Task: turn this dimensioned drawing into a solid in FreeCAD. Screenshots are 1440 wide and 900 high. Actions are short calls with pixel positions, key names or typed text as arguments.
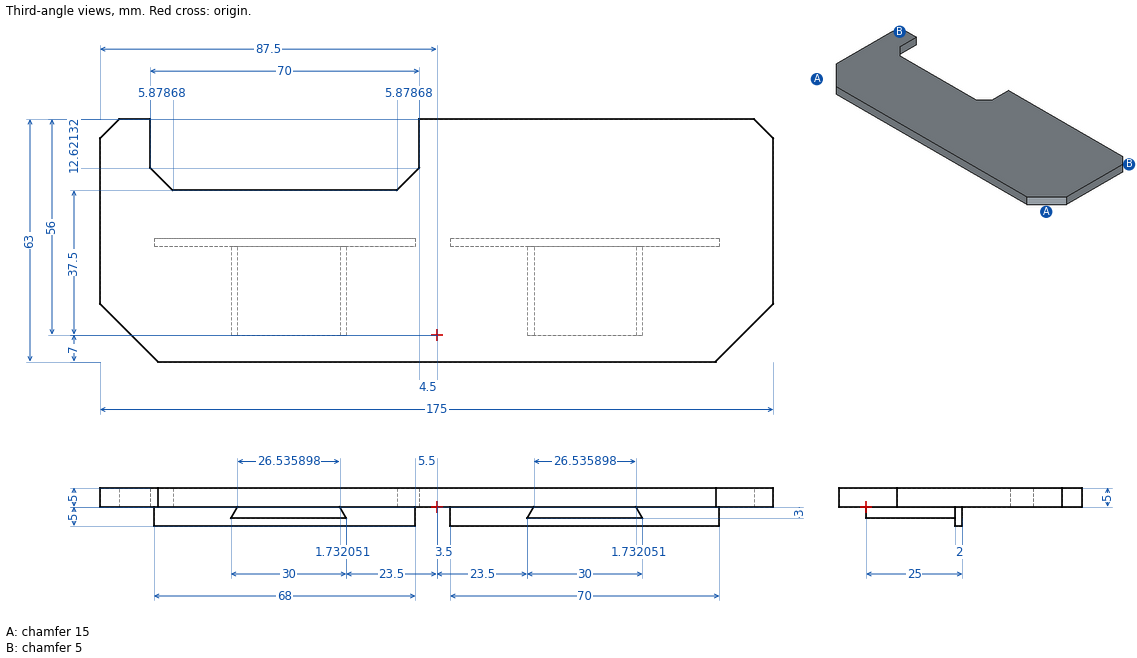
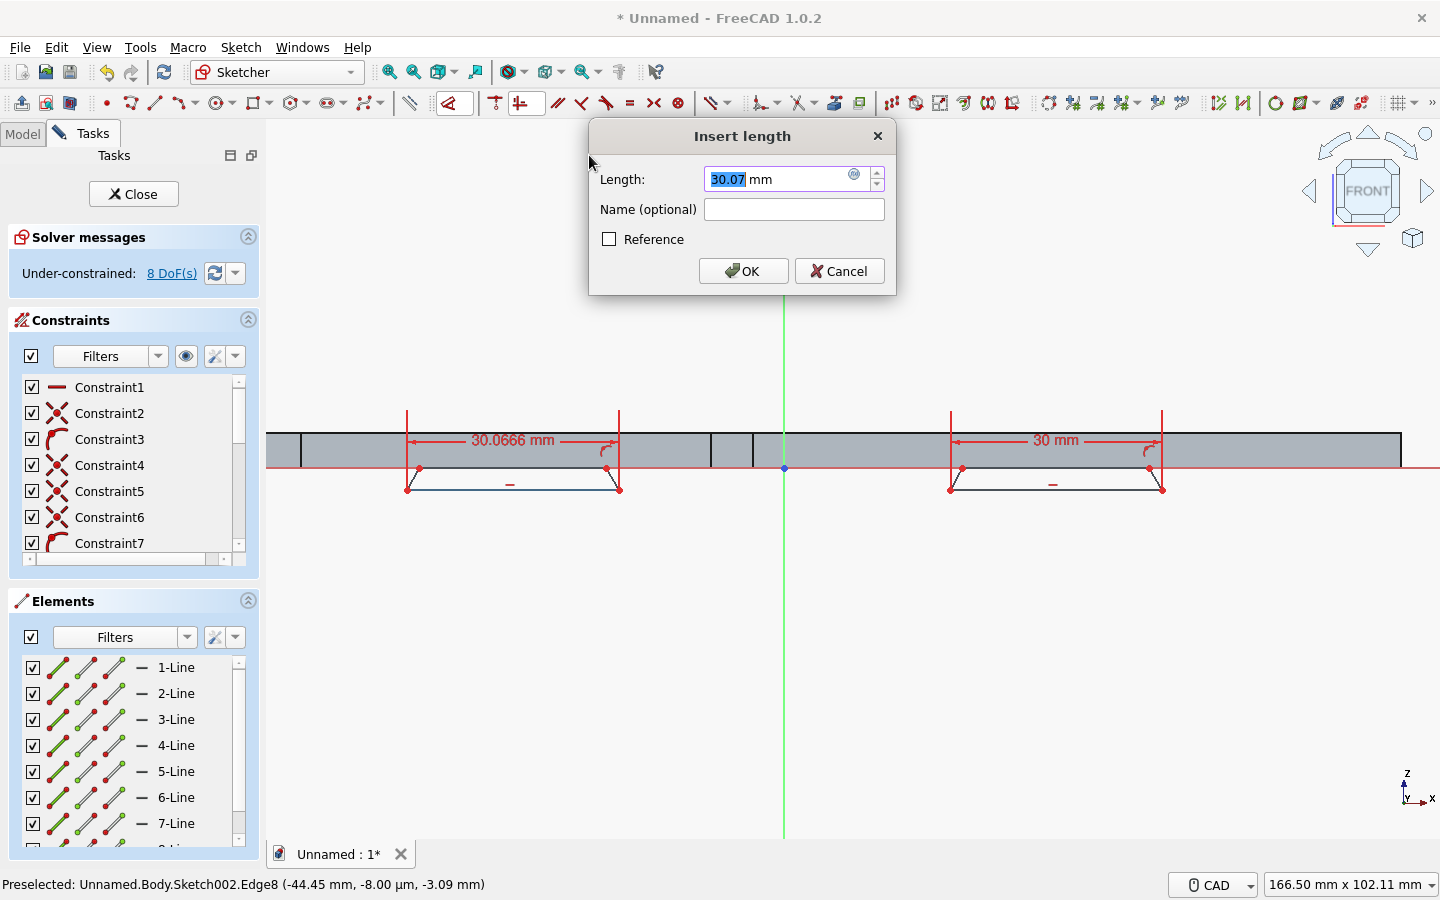
text(30)
key(Return)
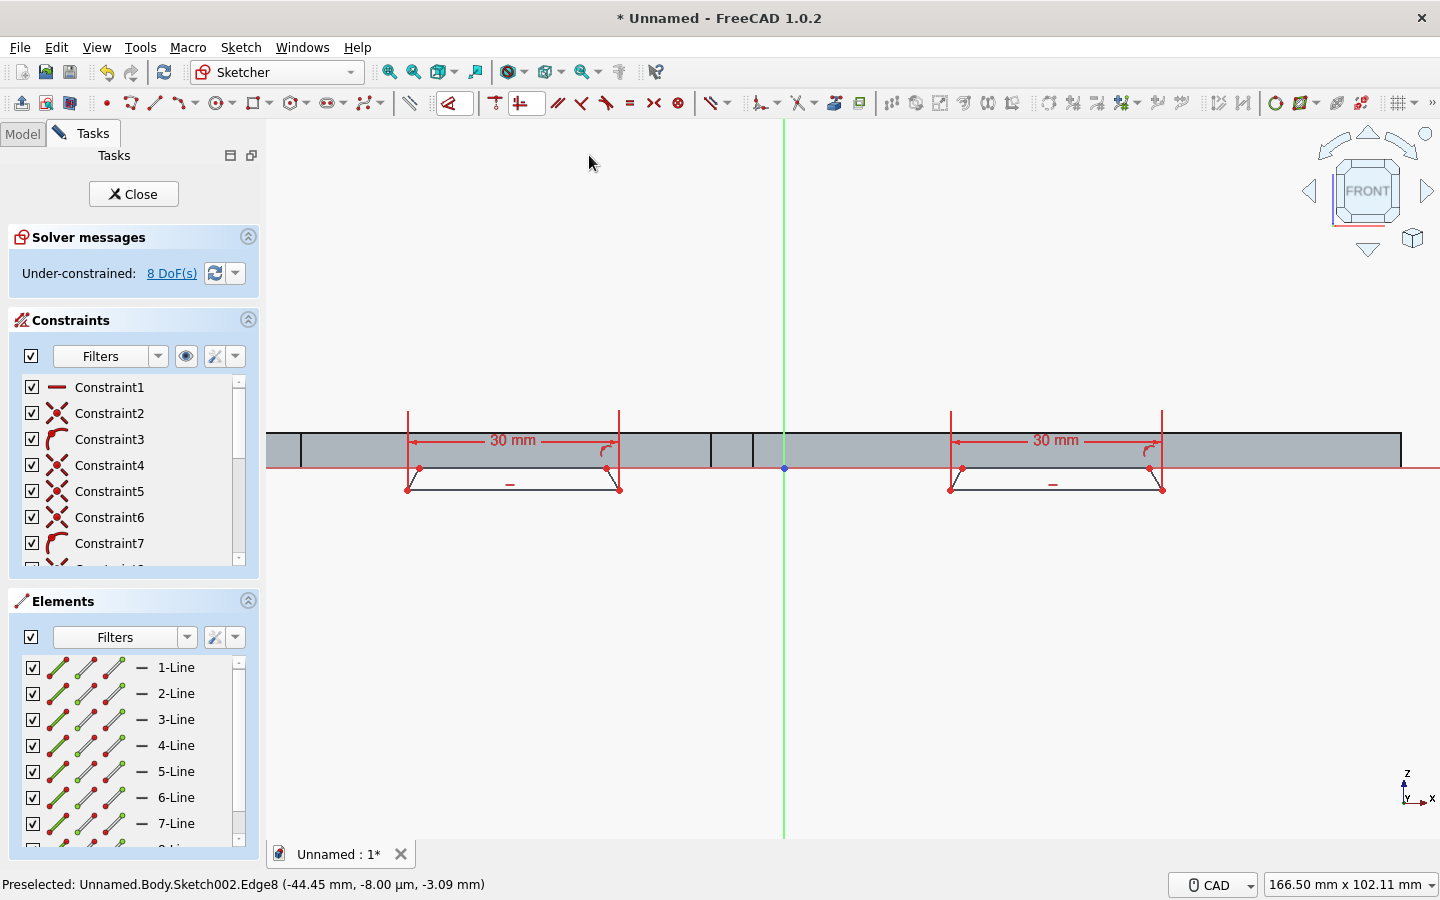
scroll(951, 490, up, 4)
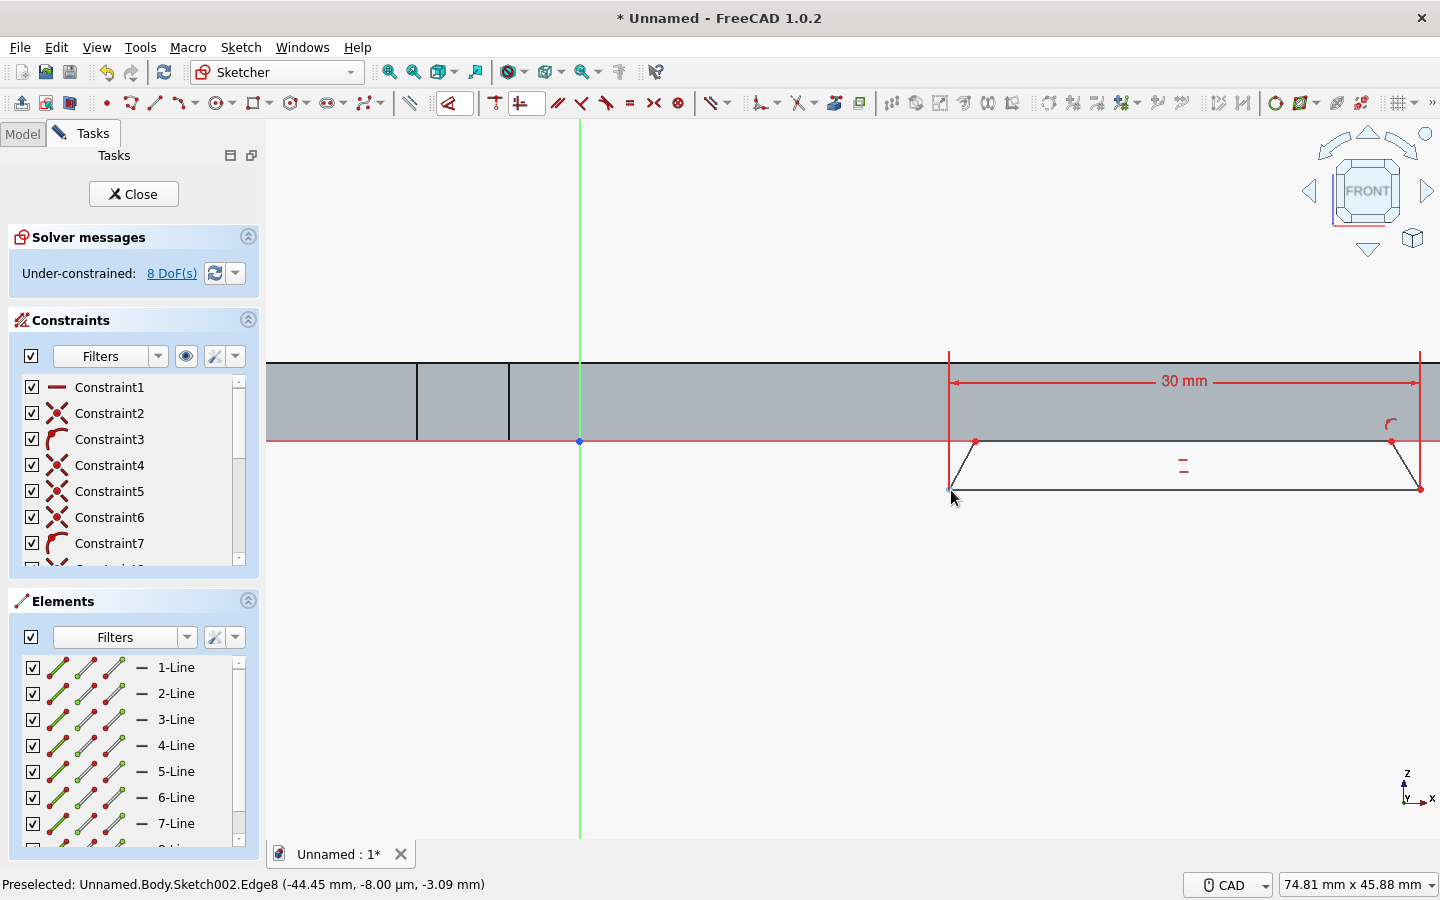
click(949, 490)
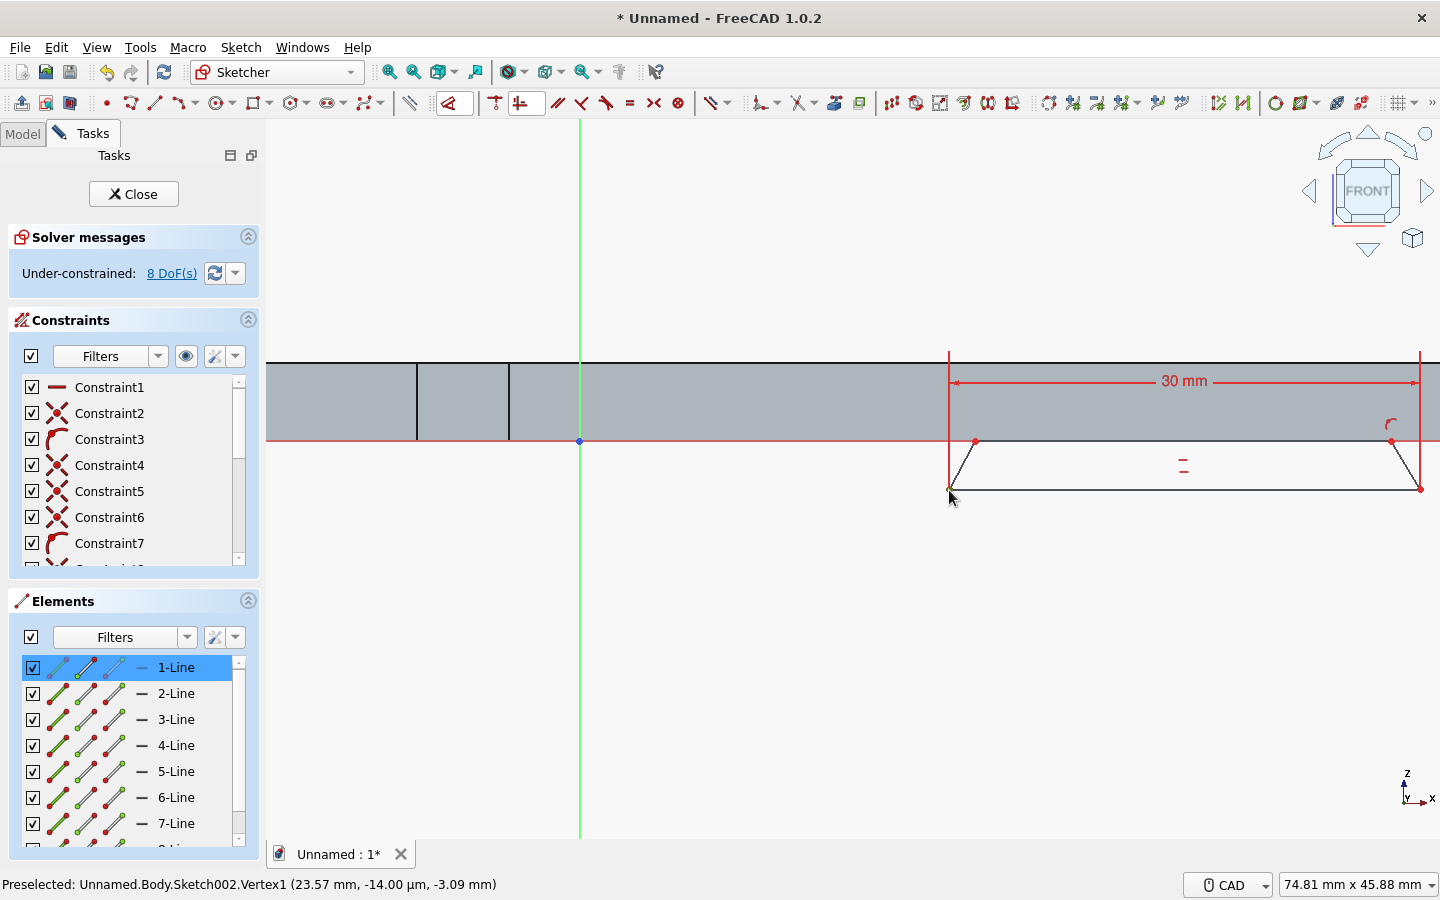
click(468, 104)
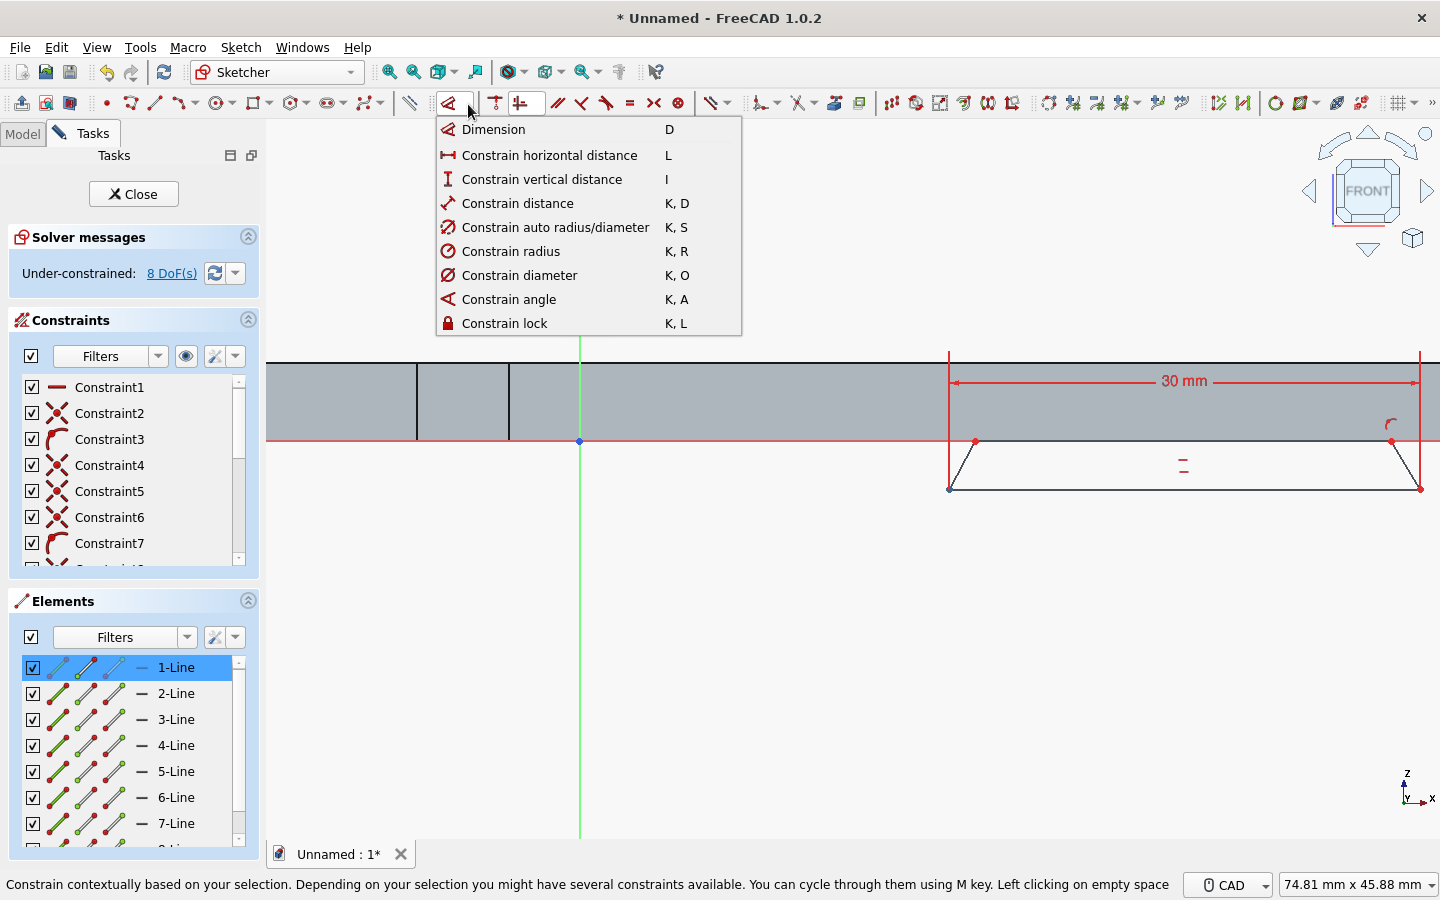
click(589, 179)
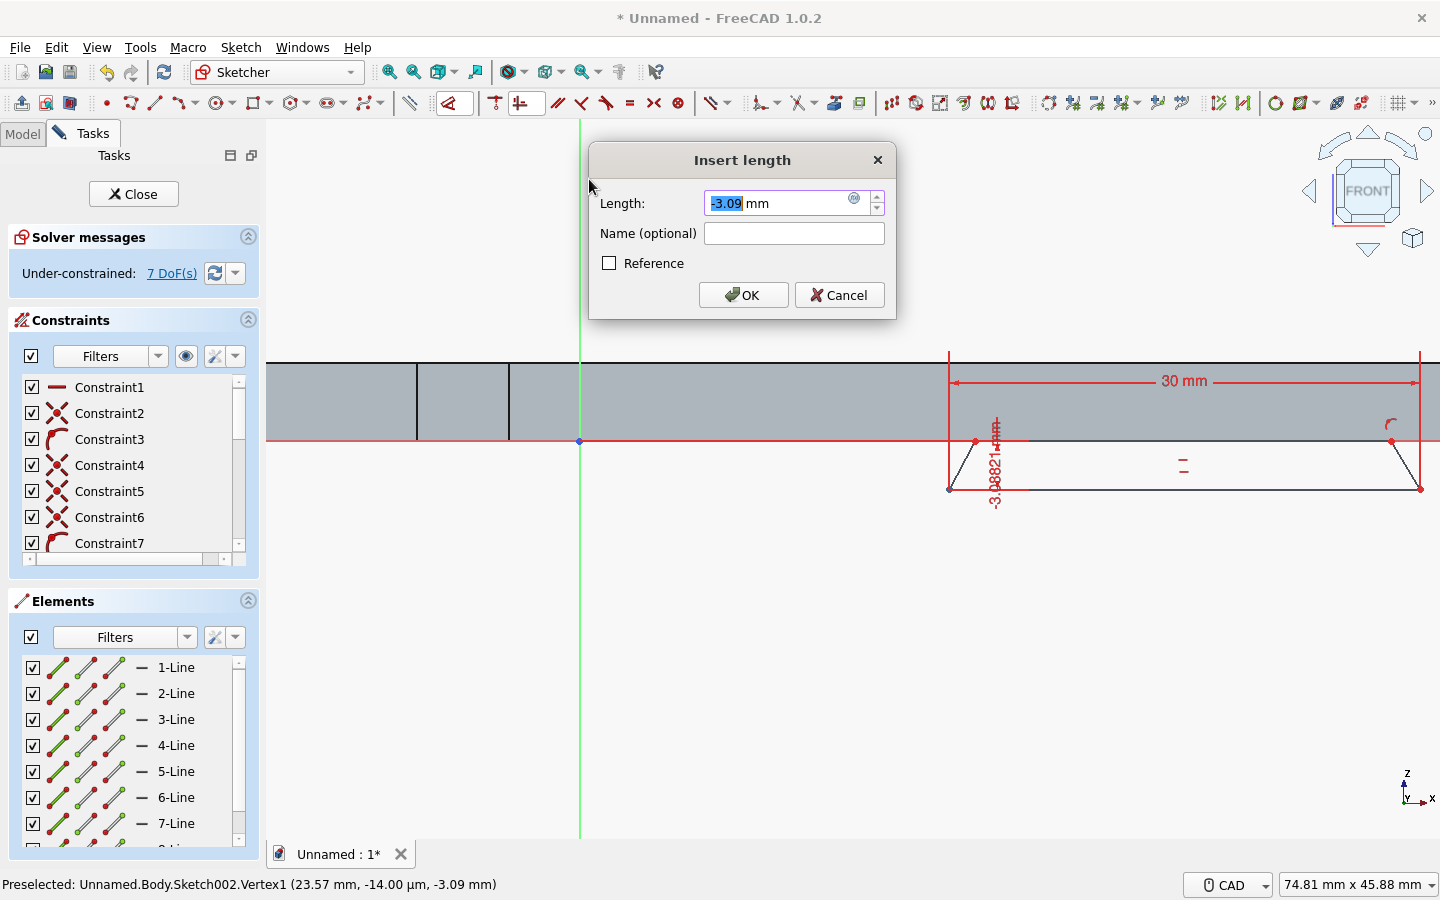
text(-3)
key(Return)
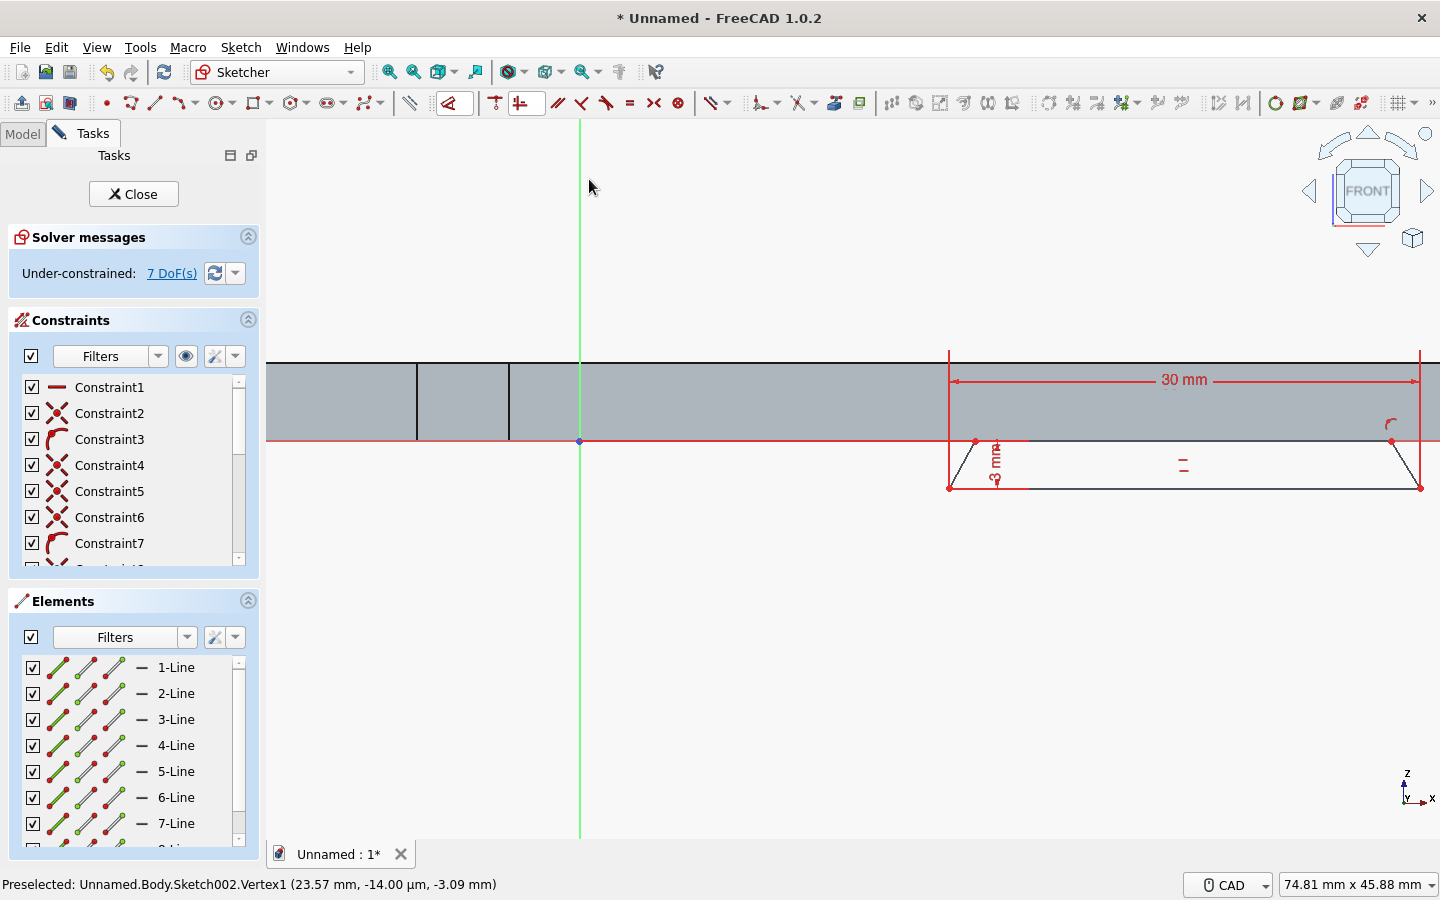
scroll(952, 490, down, 4)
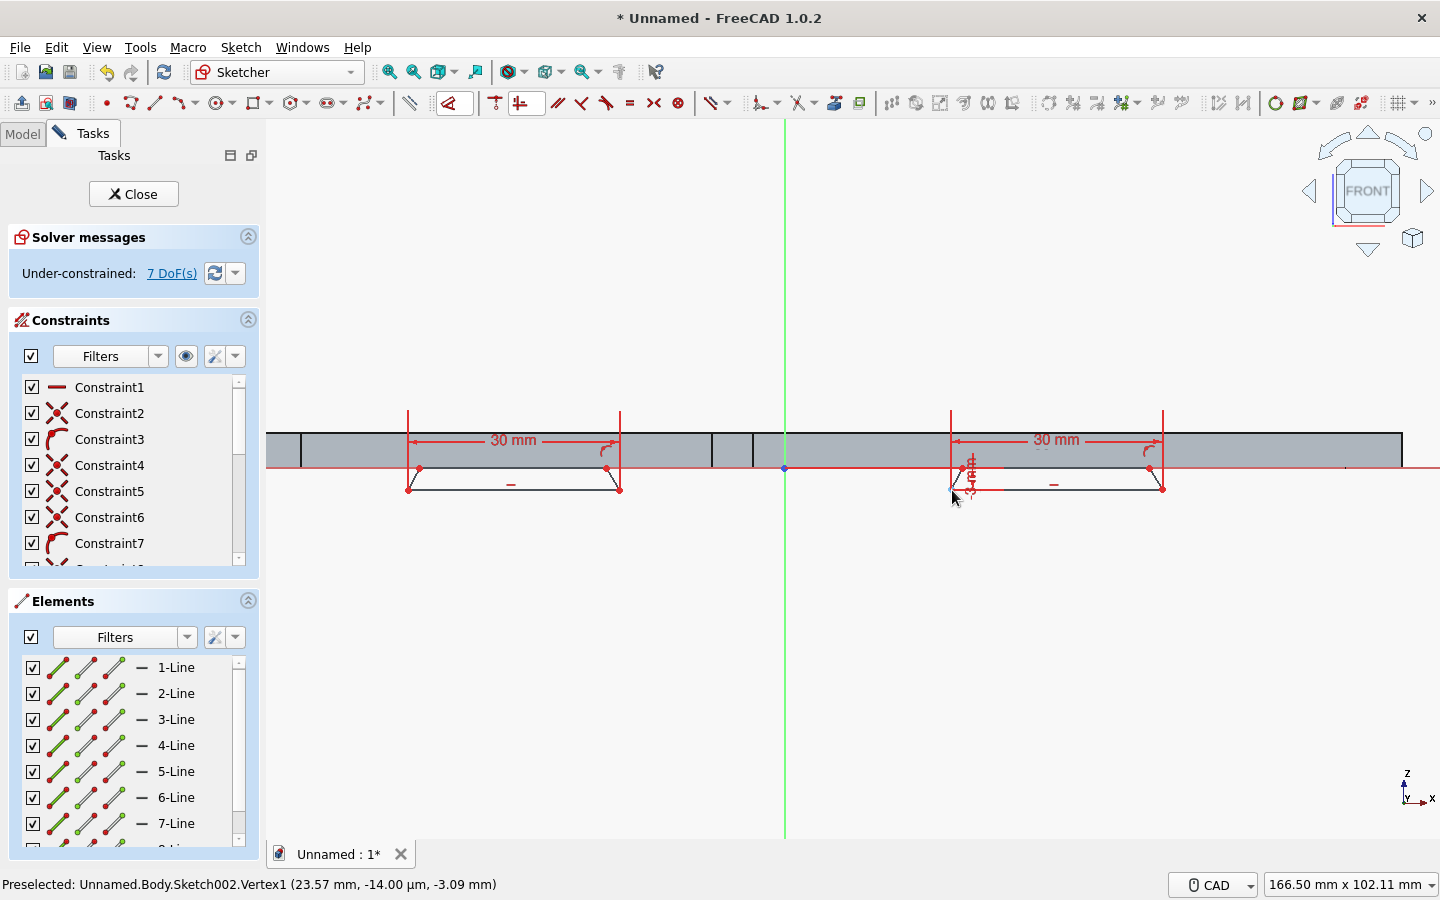
scroll(620, 490, up, 4)